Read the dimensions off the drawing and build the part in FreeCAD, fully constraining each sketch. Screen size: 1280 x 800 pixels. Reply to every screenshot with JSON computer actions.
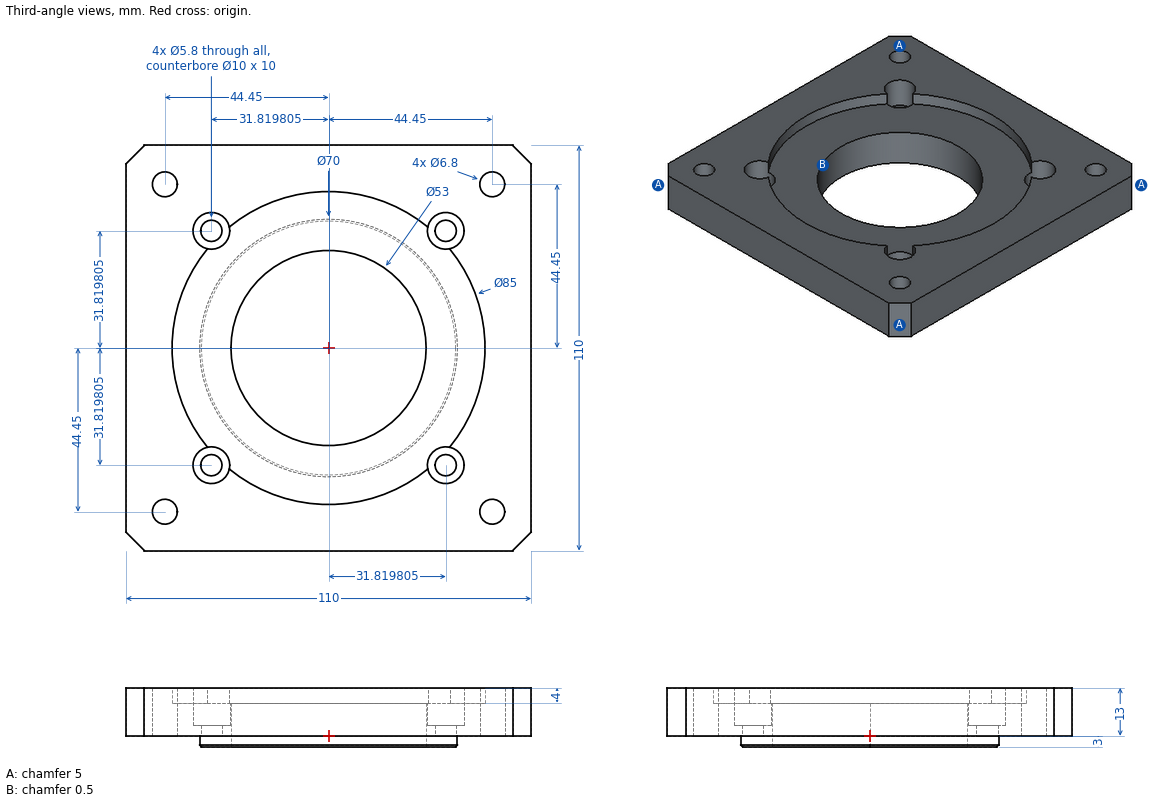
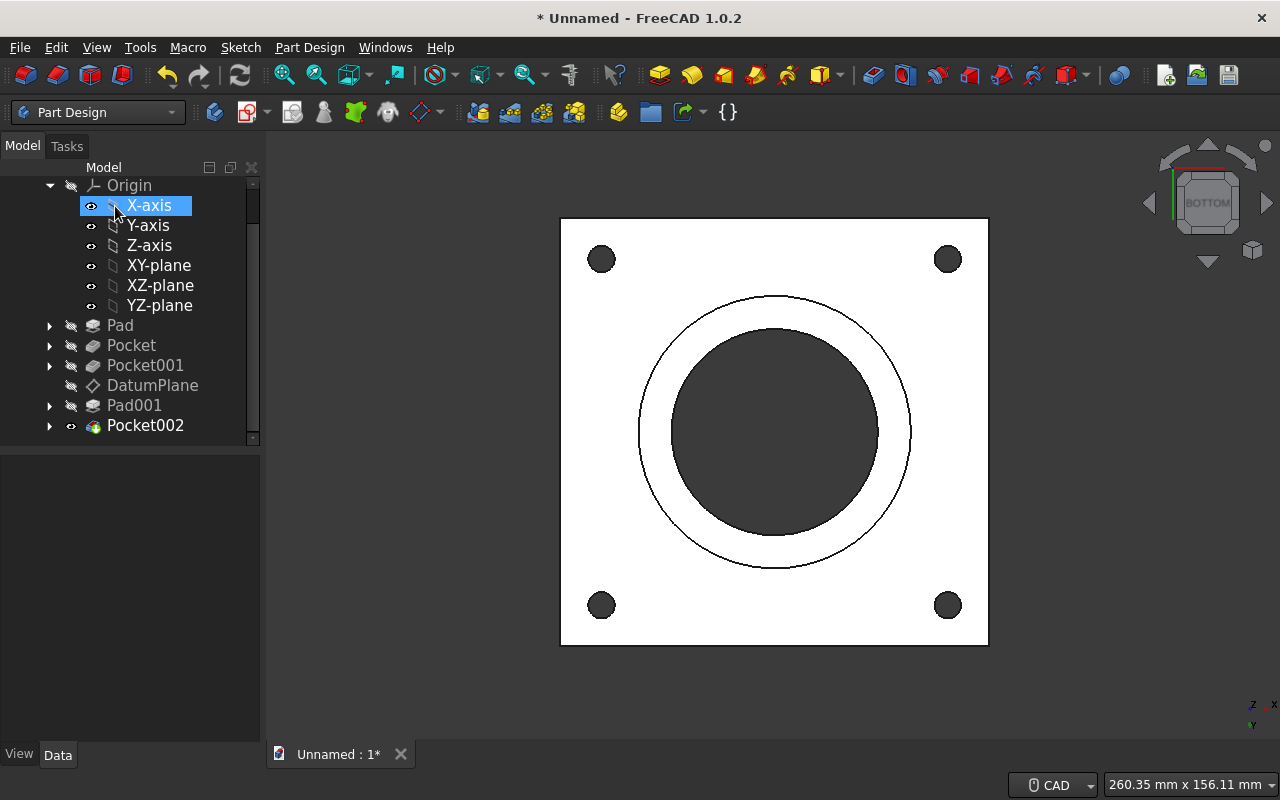
{"action": "key", "text": "0"}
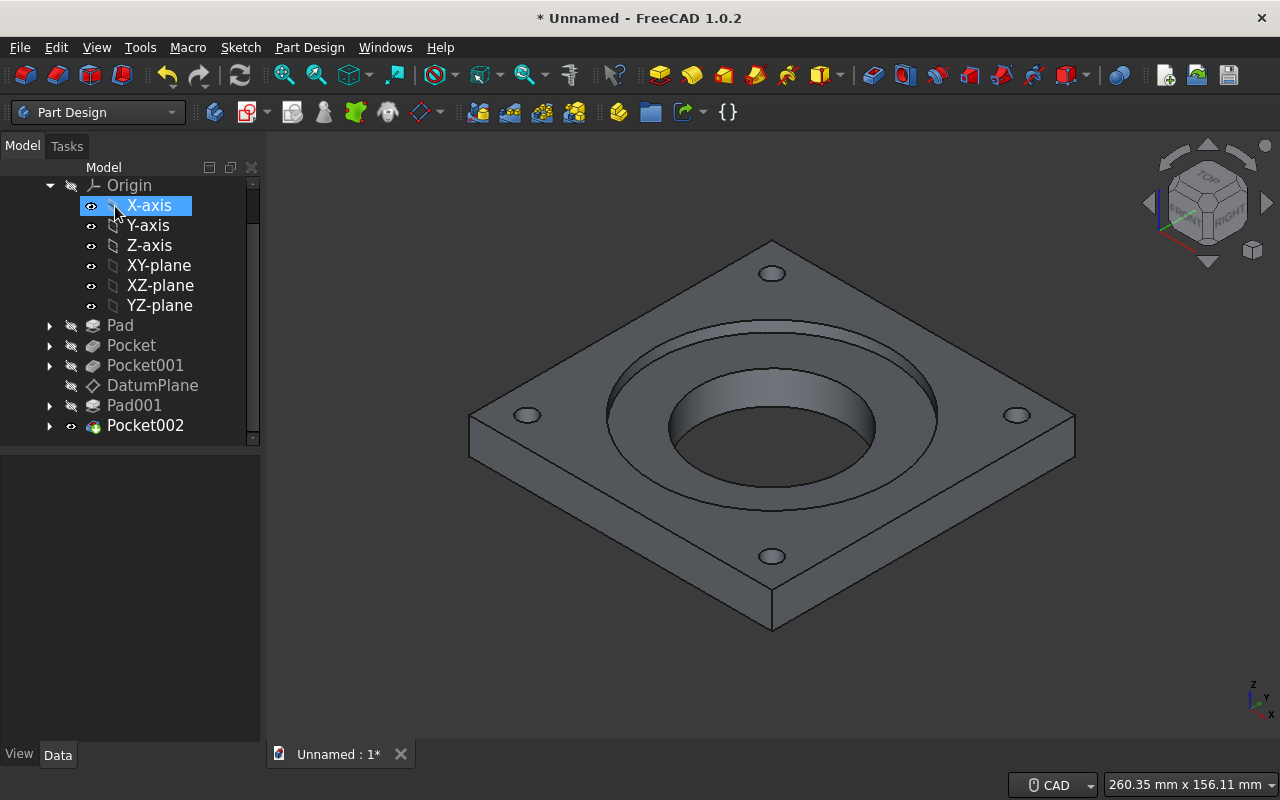
{"action": "left_click", "coordinate": [772, 610]}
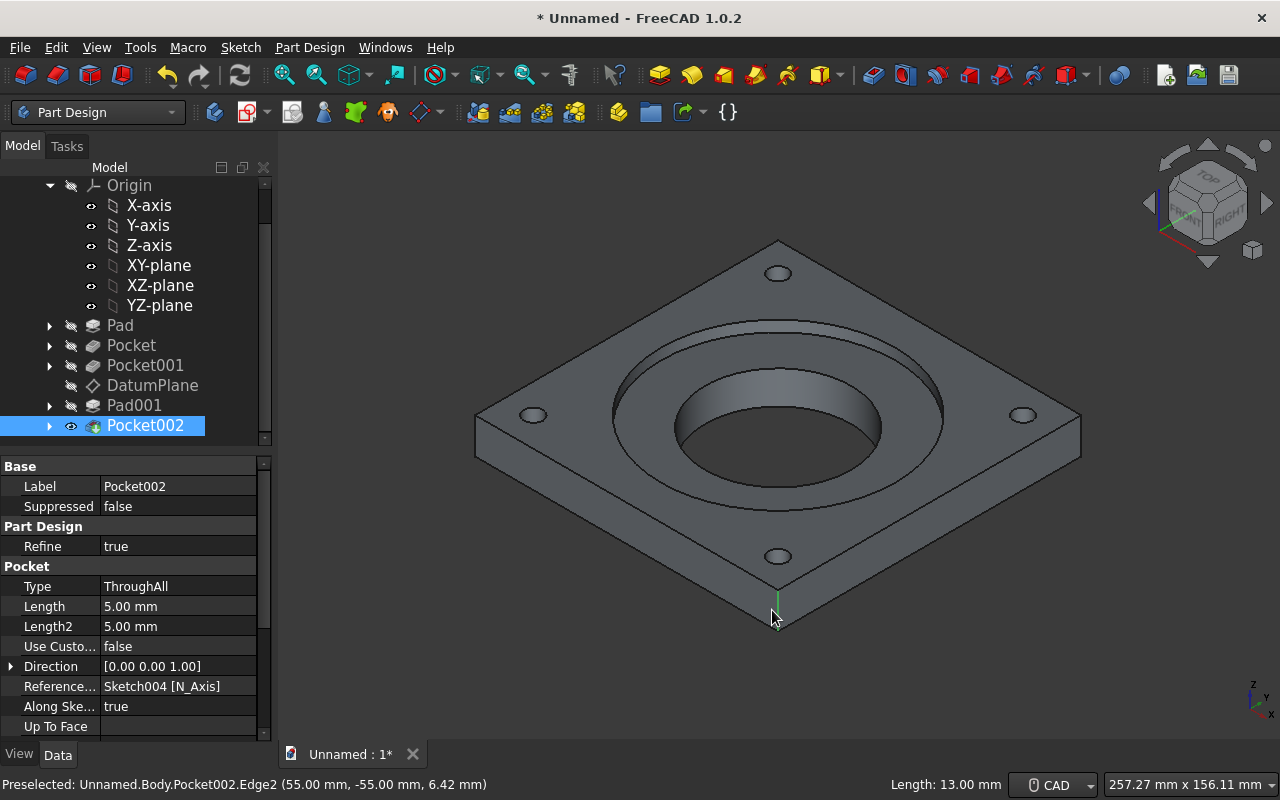
{"action": "key", "text": "2"}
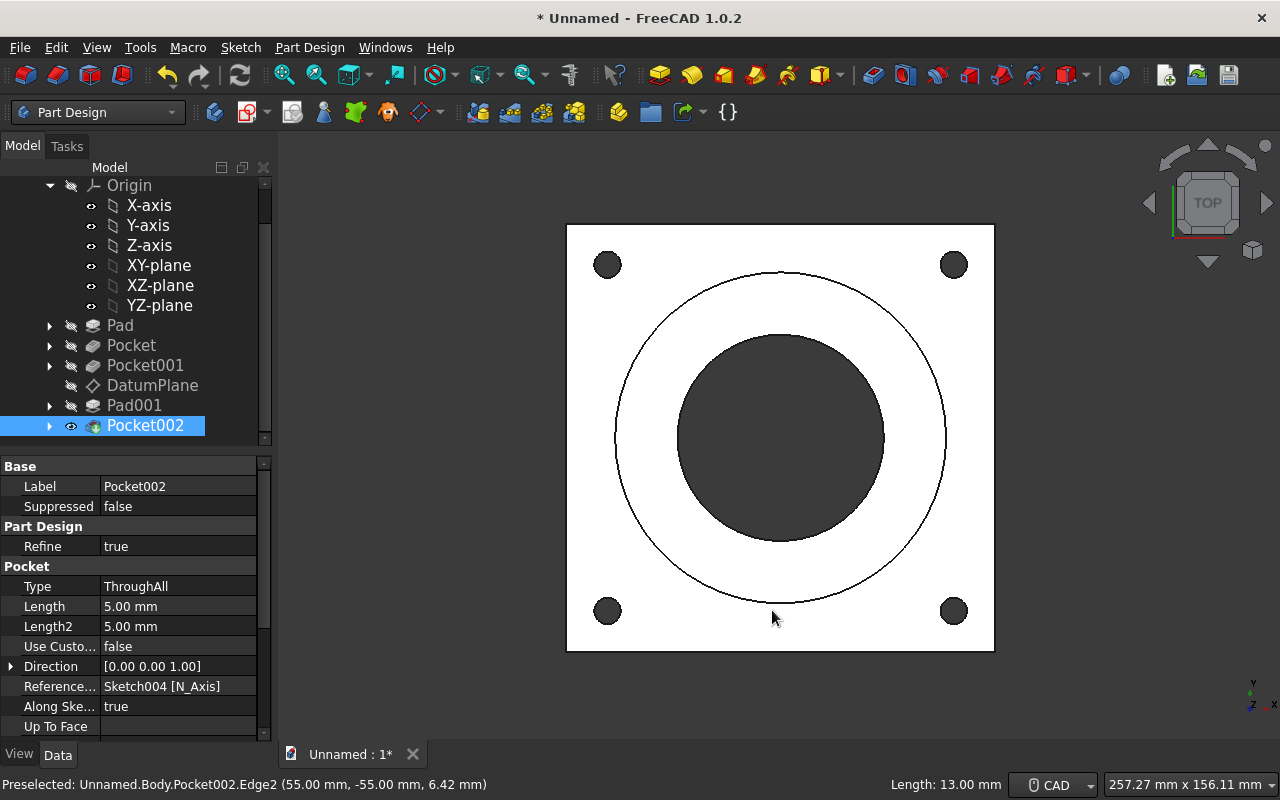
{"action": "key", "text": "1"}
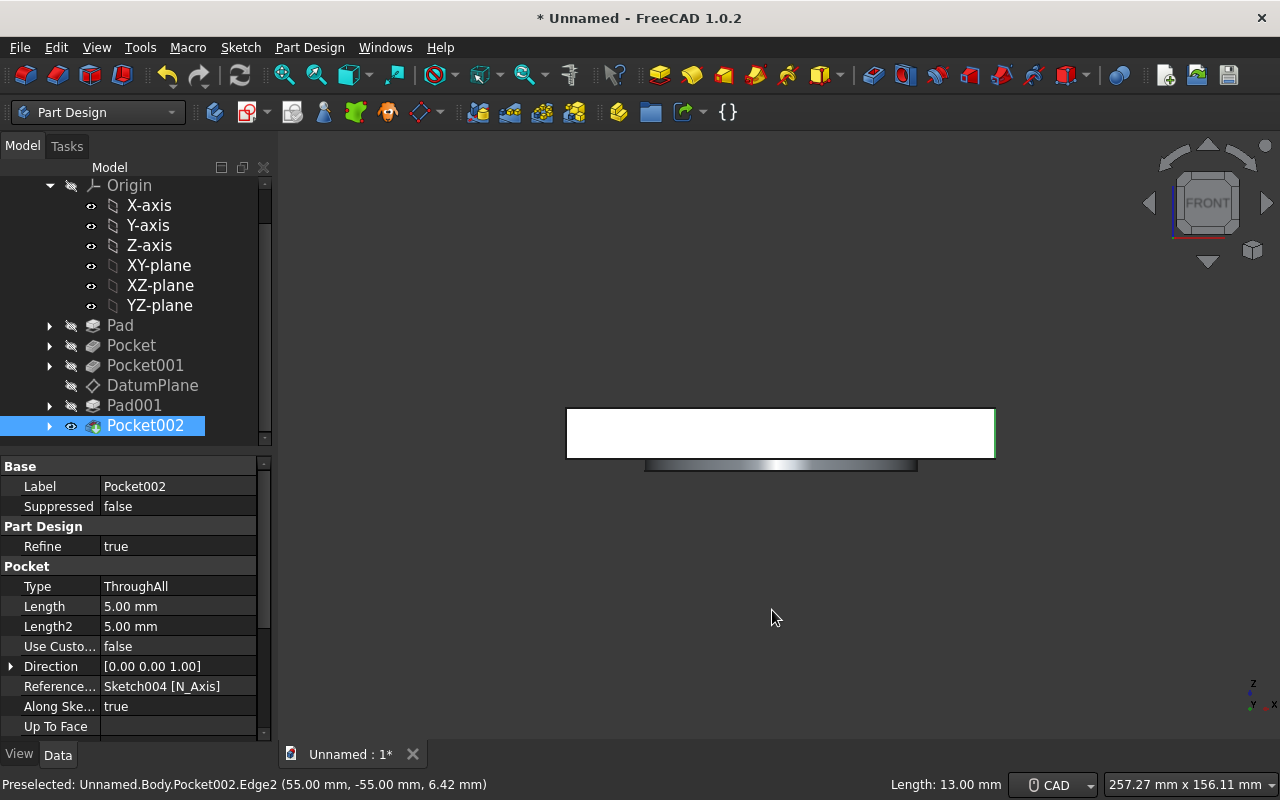
{"action": "key", "text": "v f"}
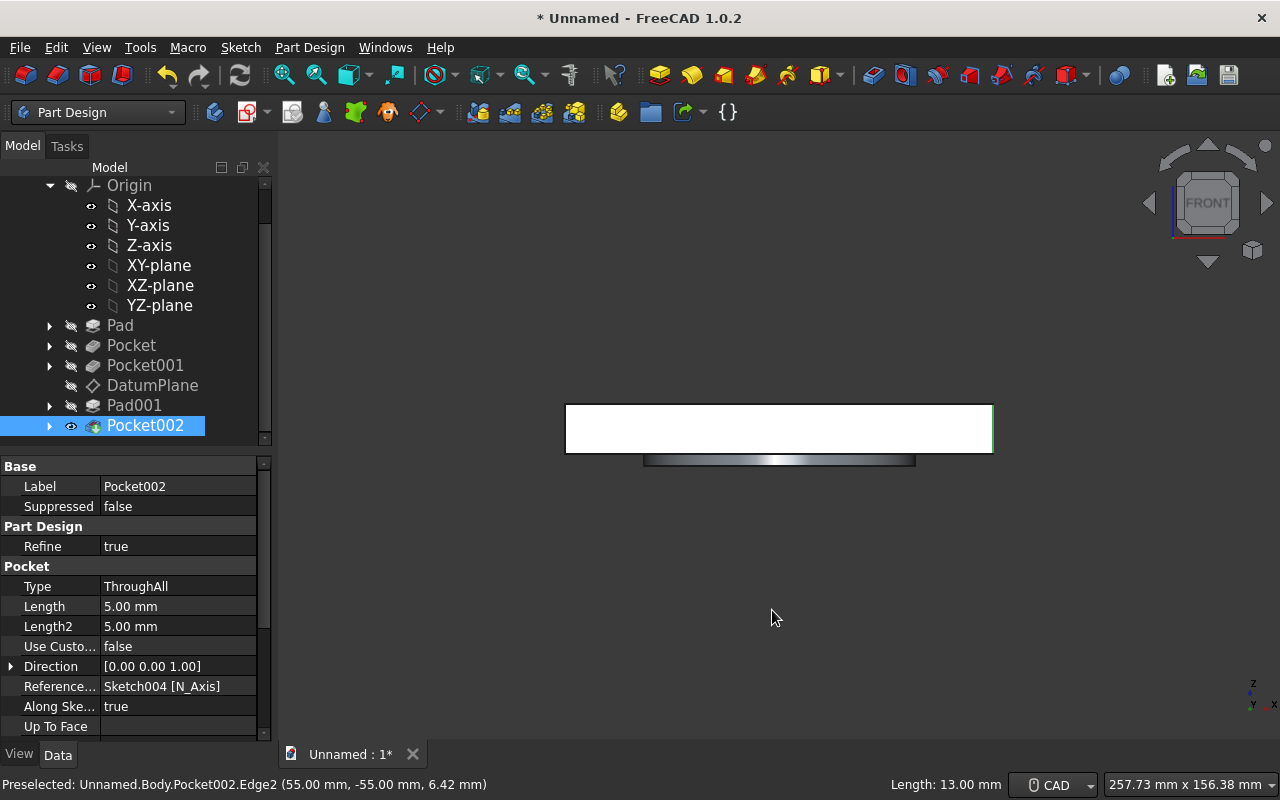
{"action": "left_click", "coordinate": [565, 428], "text": "ctrl"}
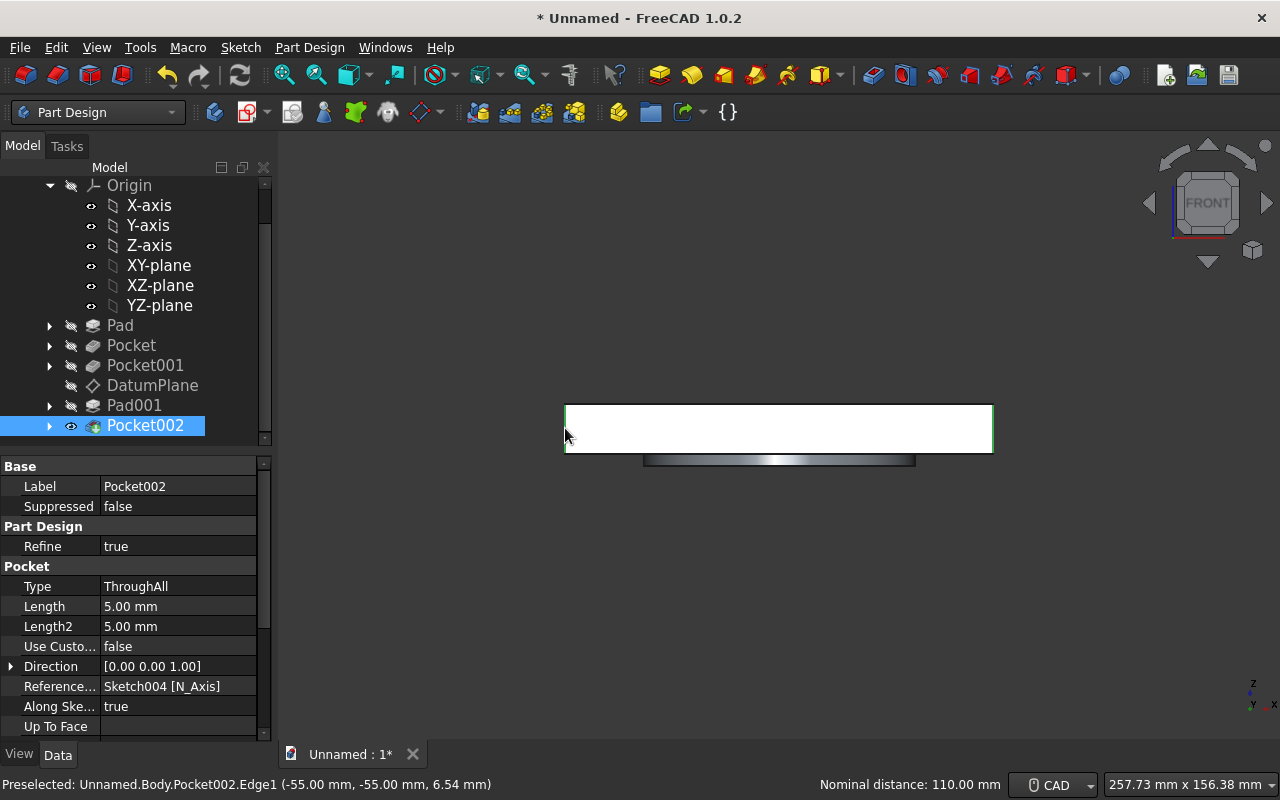
{"action": "key", "text": "3"}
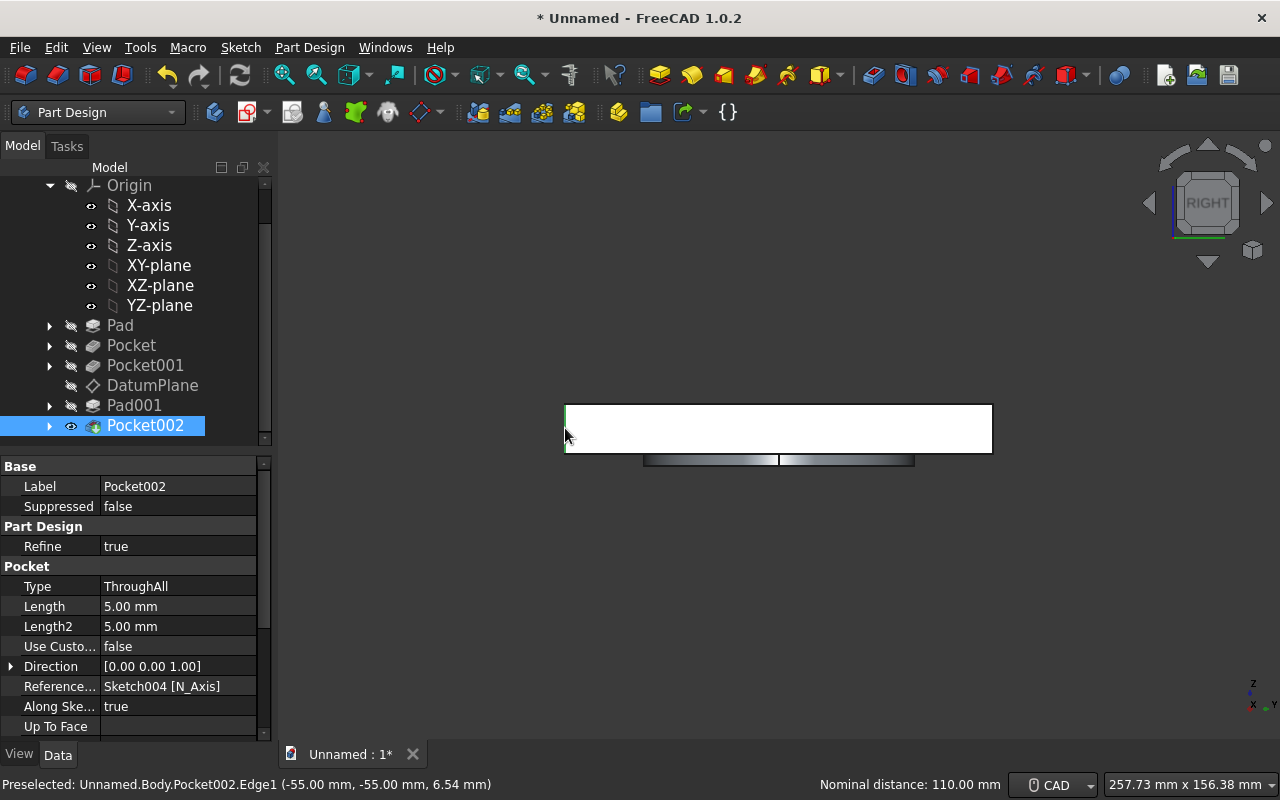
{"action": "left_click", "coordinate": [286, 76]}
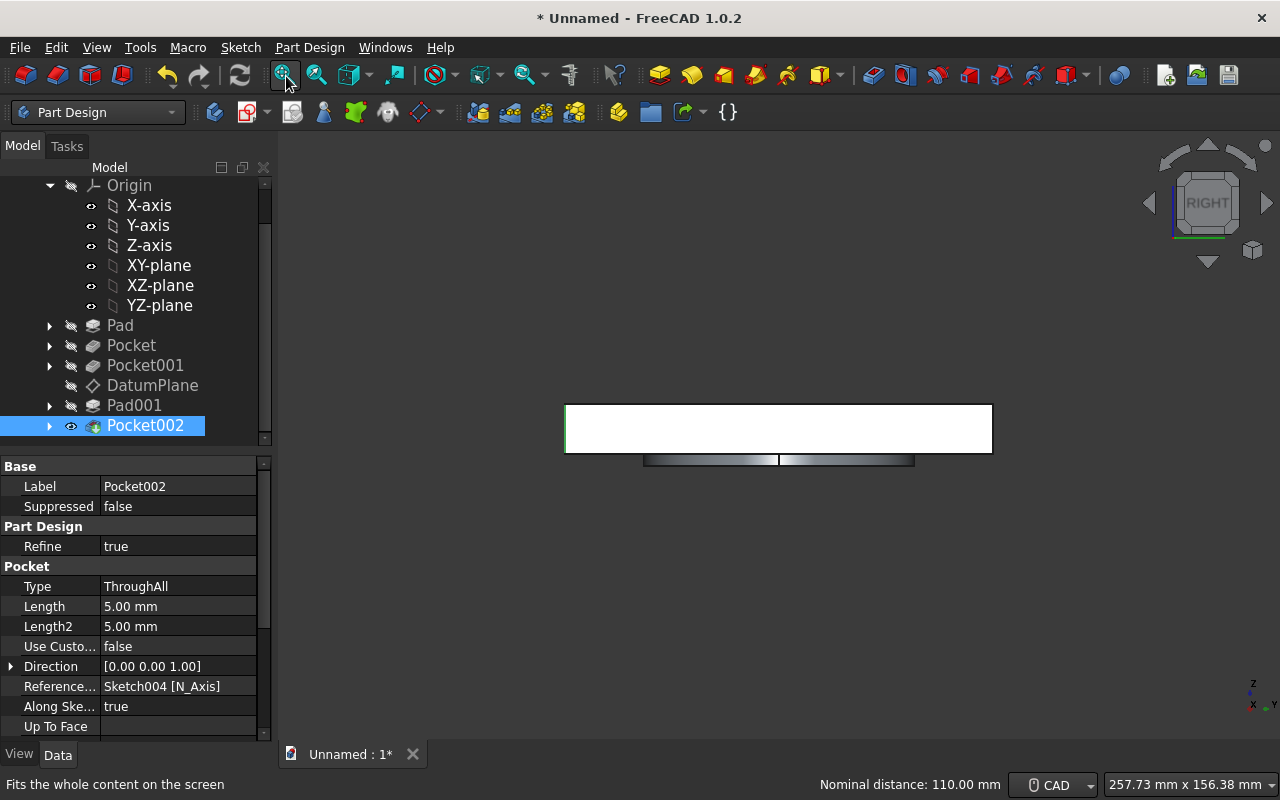
{"action": "left_click", "coordinate": [993, 428], "text": "ctrl"}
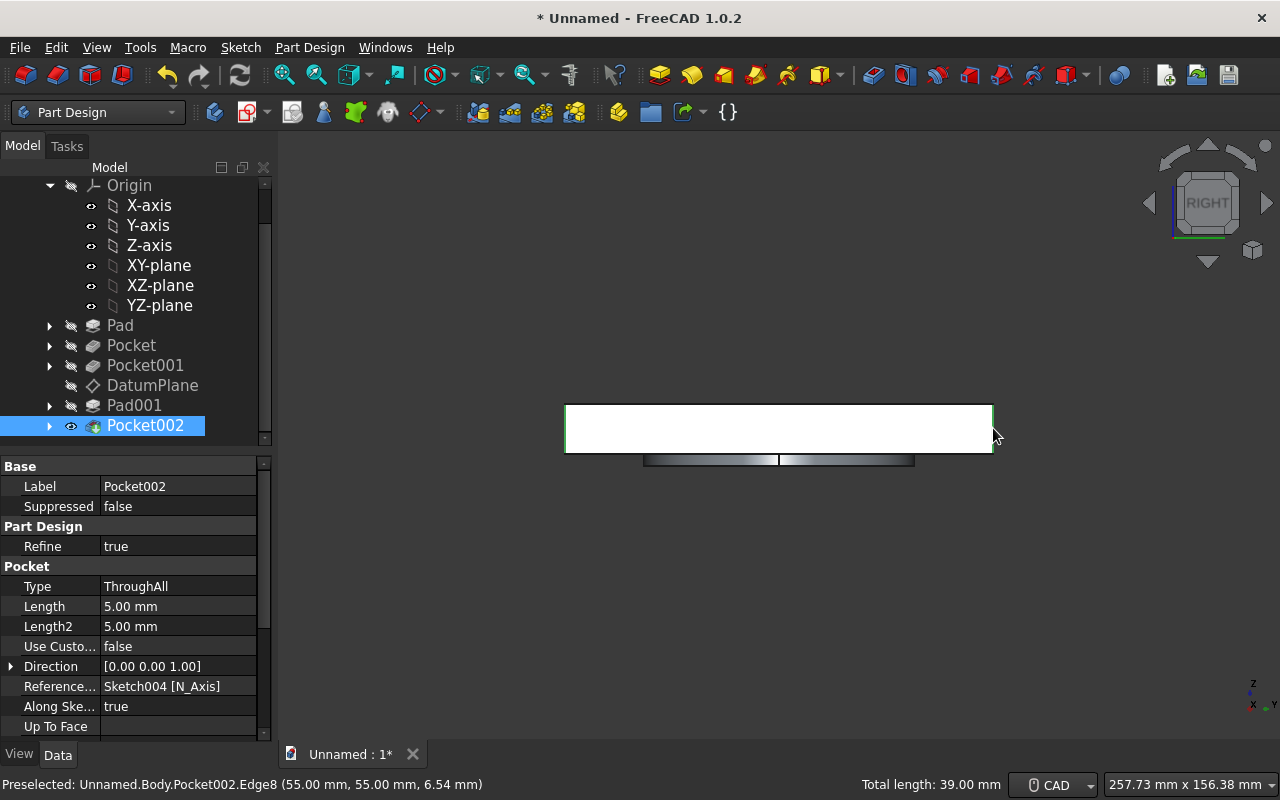
{"action": "key", "text": "5"}